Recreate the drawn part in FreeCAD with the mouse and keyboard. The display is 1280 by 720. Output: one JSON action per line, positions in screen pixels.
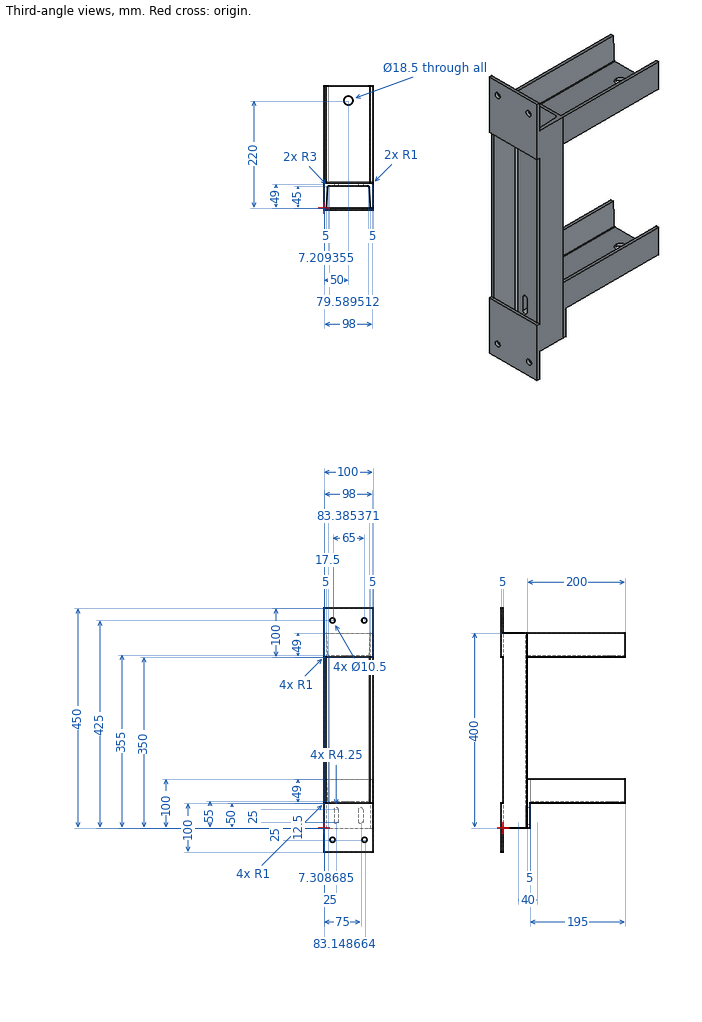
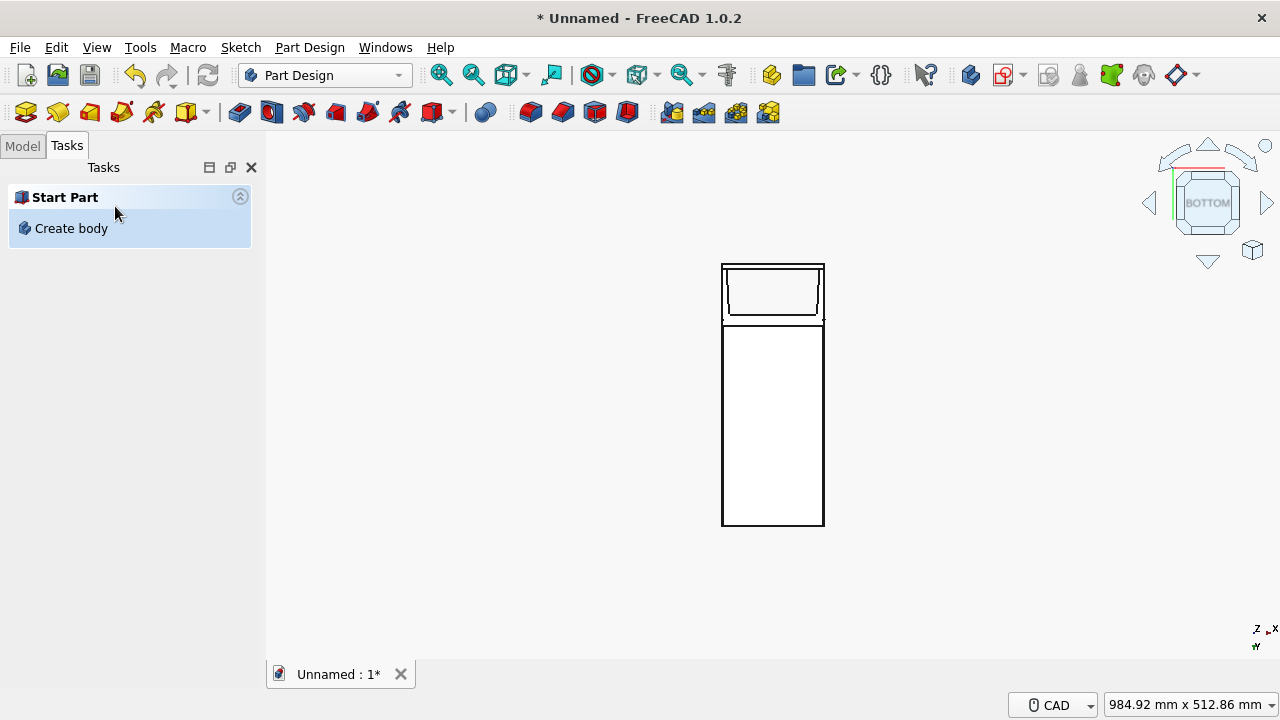
{"action": "left_click", "coordinate": [773, 454]}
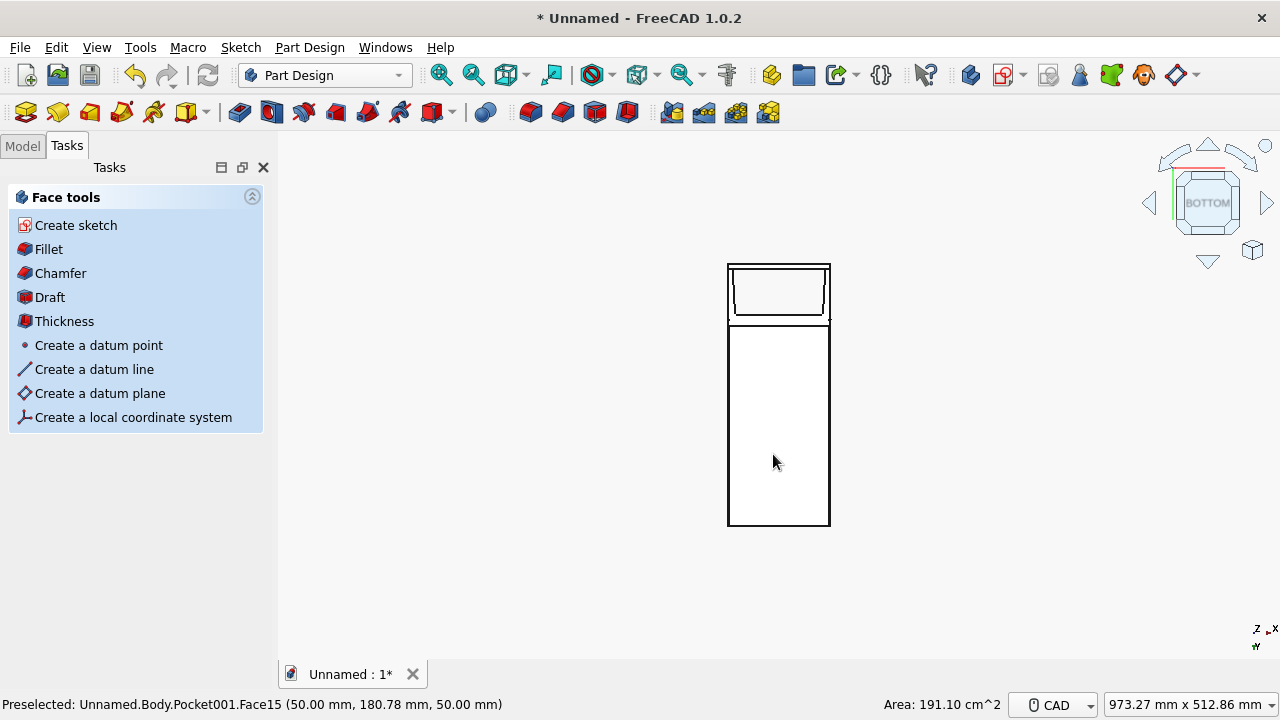
{"action": "left_click", "coordinate": [1004, 76]}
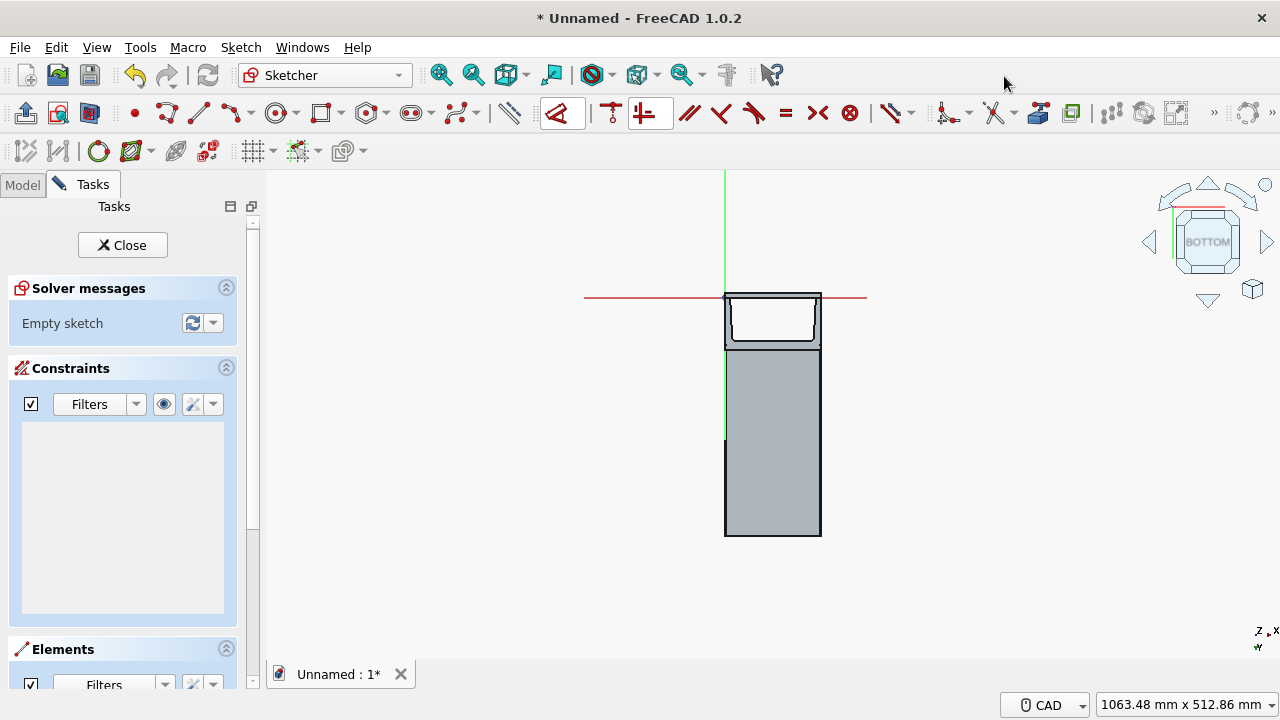
{"action": "key", "text": "q s"}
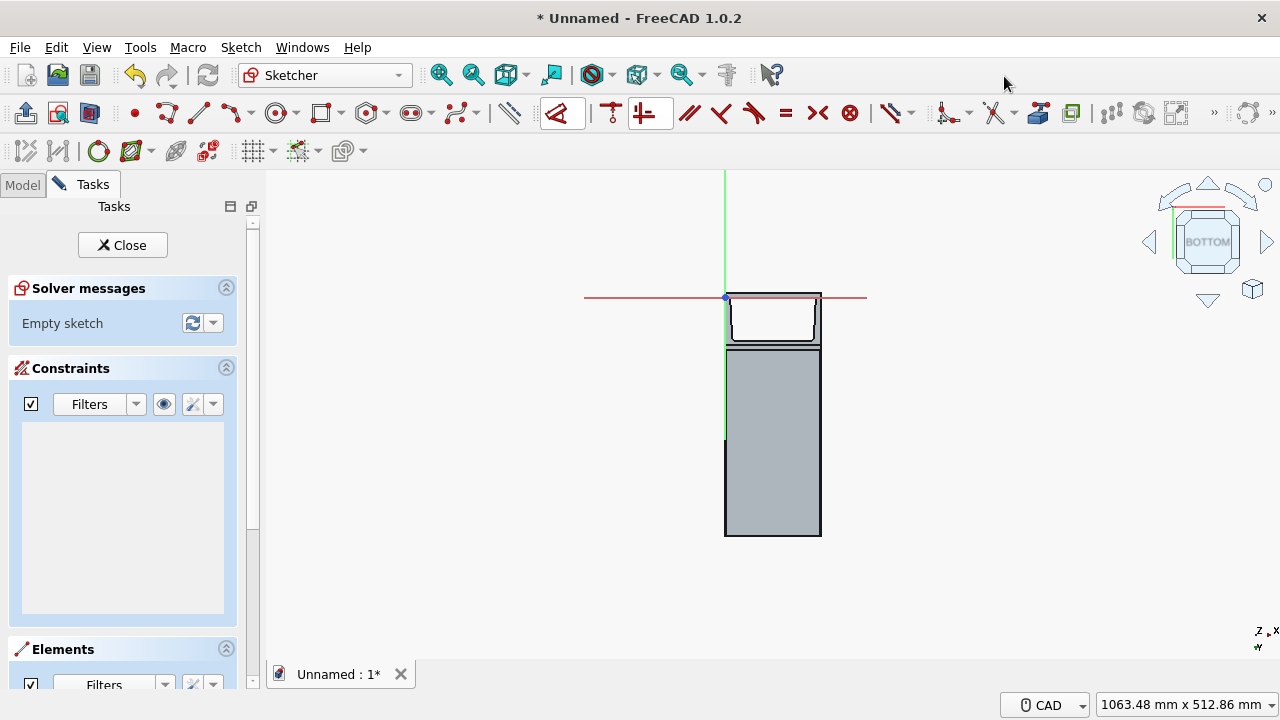
{"action": "scroll", "coordinate": [777, 513], "scroll_direction": "up", "scroll_amount": 14}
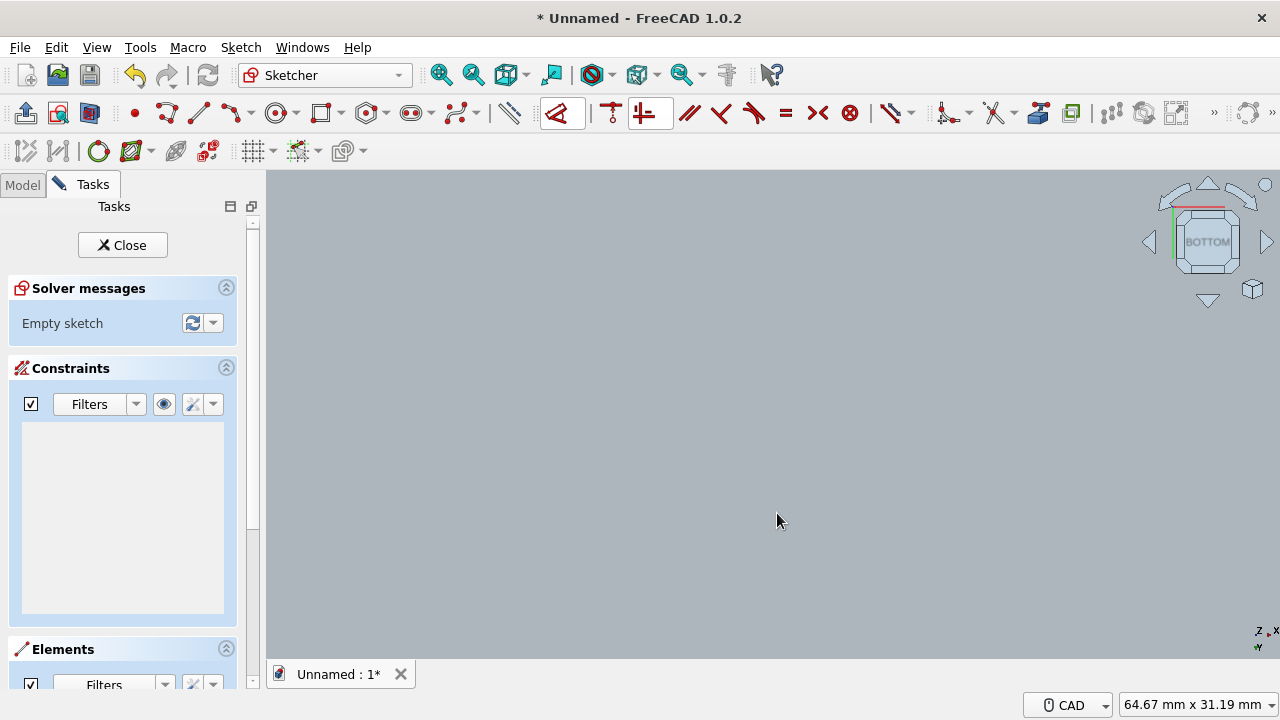
{"action": "left_click", "coordinate": [276, 114]}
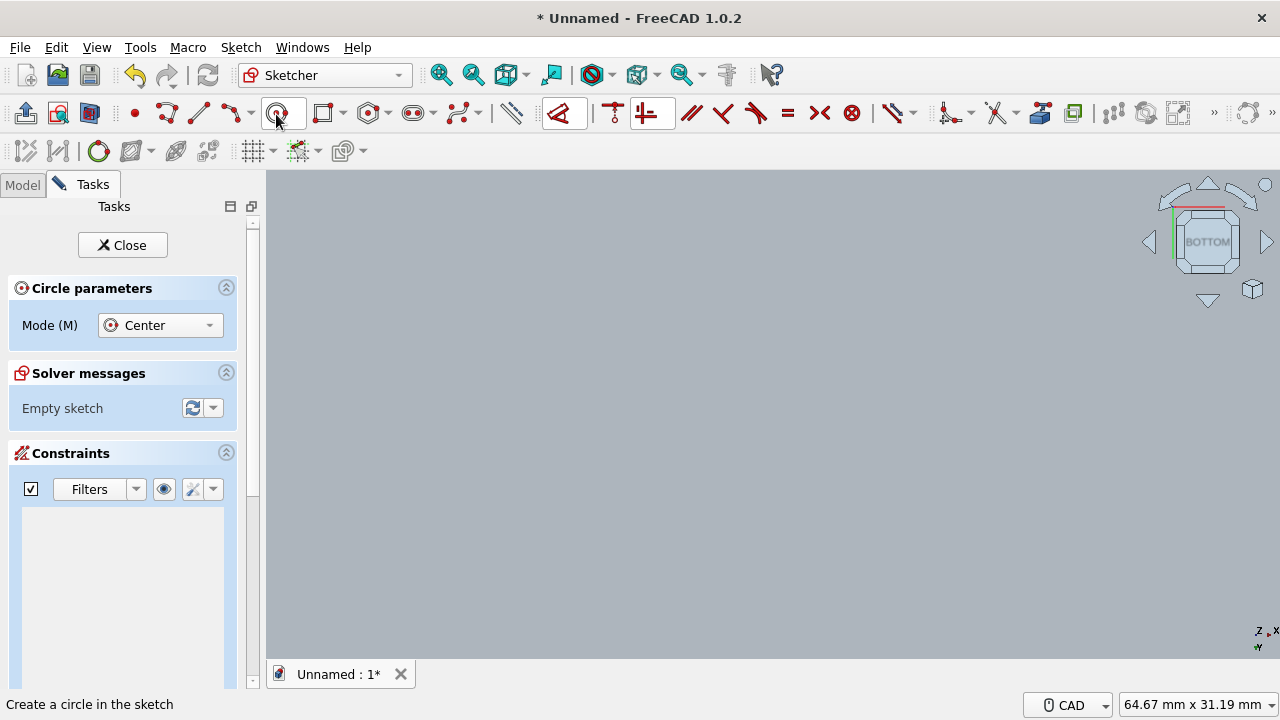
{"action": "left_click", "coordinate": [703, 411]}
{"action": "left_click", "coordinate": [806, 309]}
{"action": "key", "text": "Escape"}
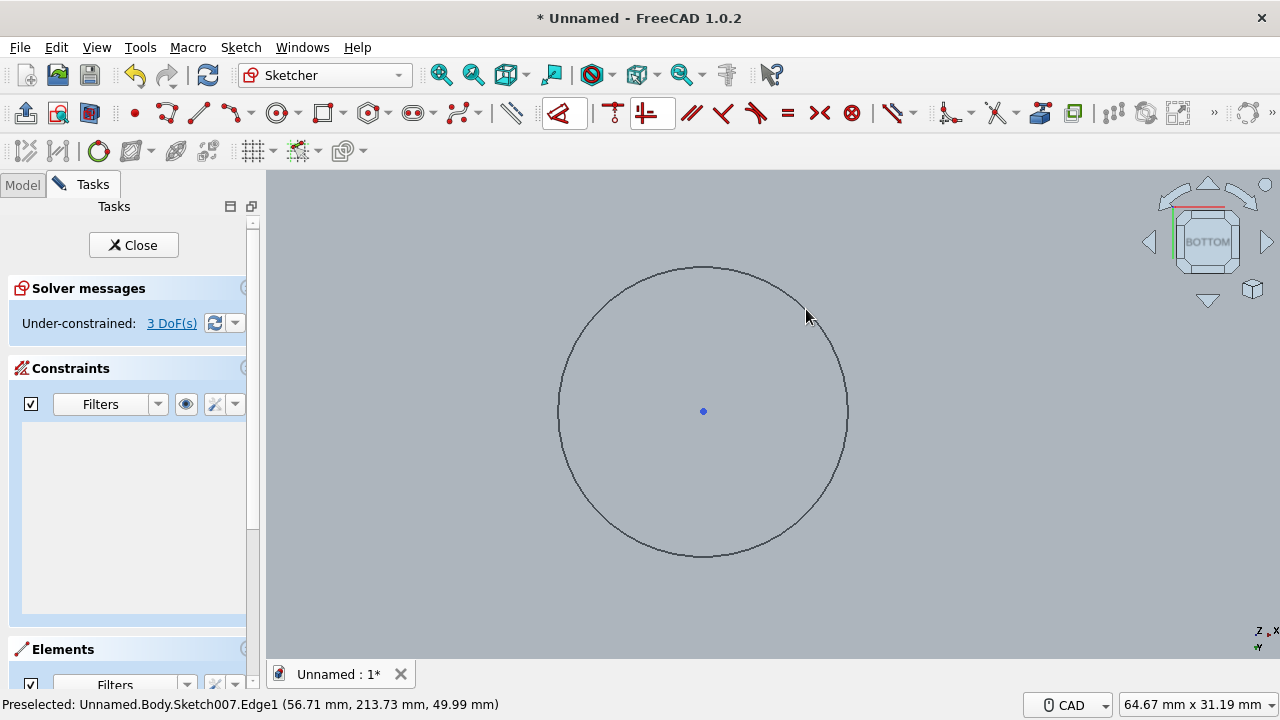
{"action": "left_click", "coordinate": [805, 309]}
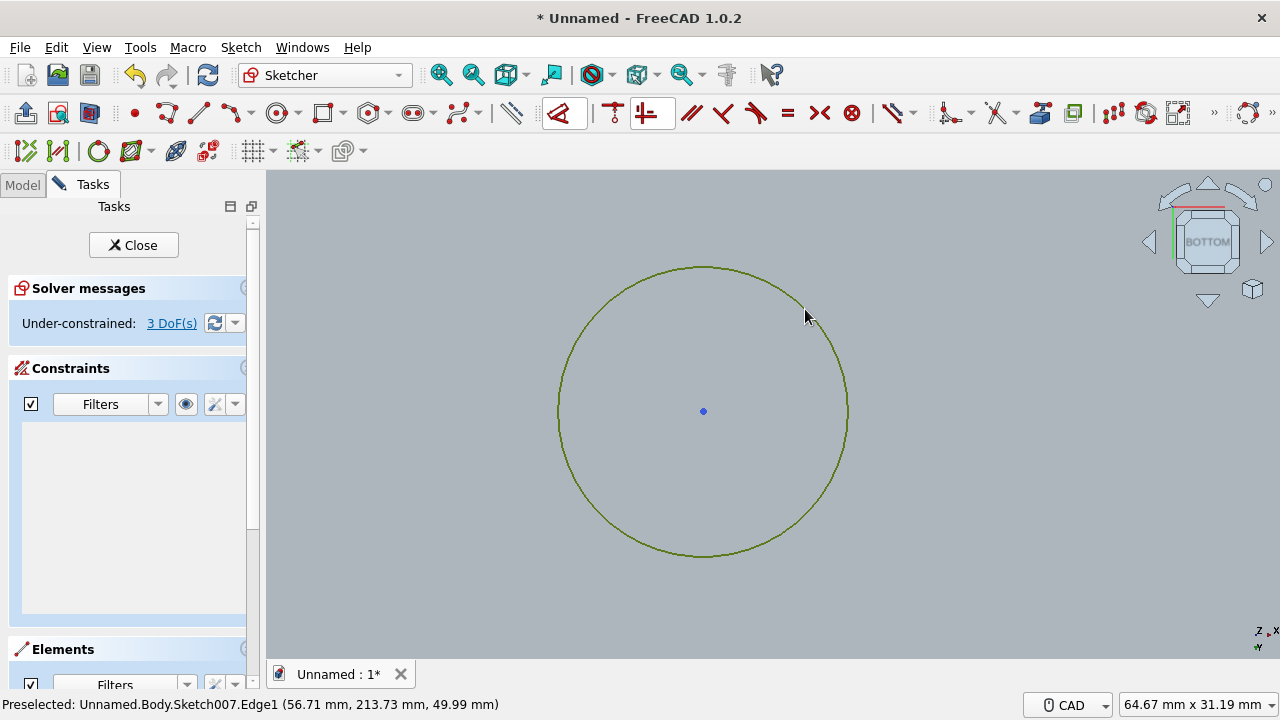
{"action": "key", "text": "k o"}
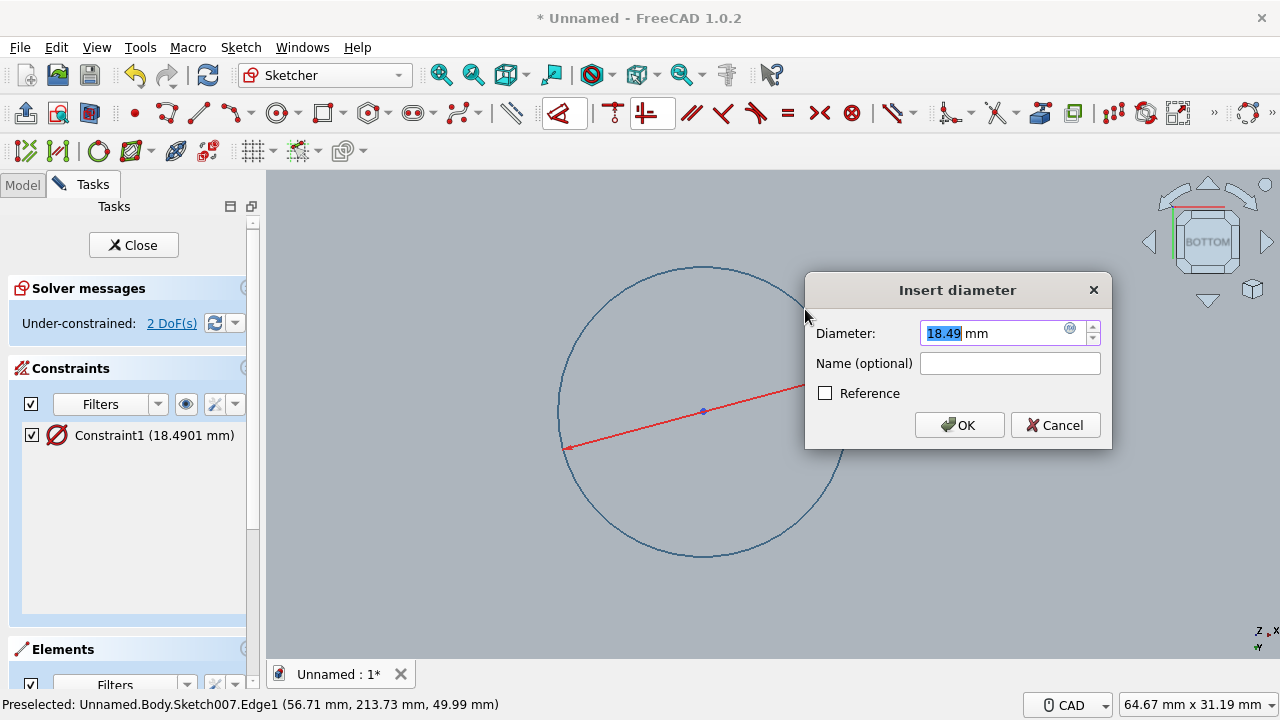
{"action": "type", "text": "18.5"}
{"action": "key", "text": "Return"}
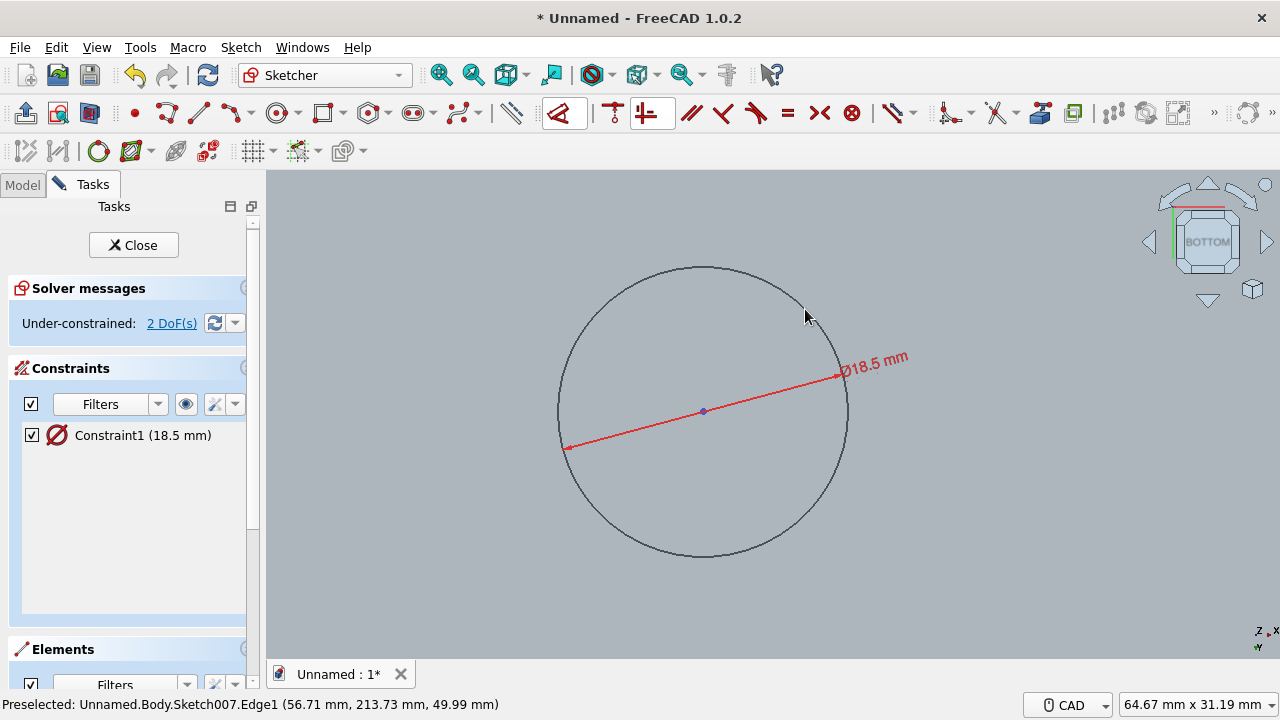
{"action": "left_click", "coordinate": [703, 412]}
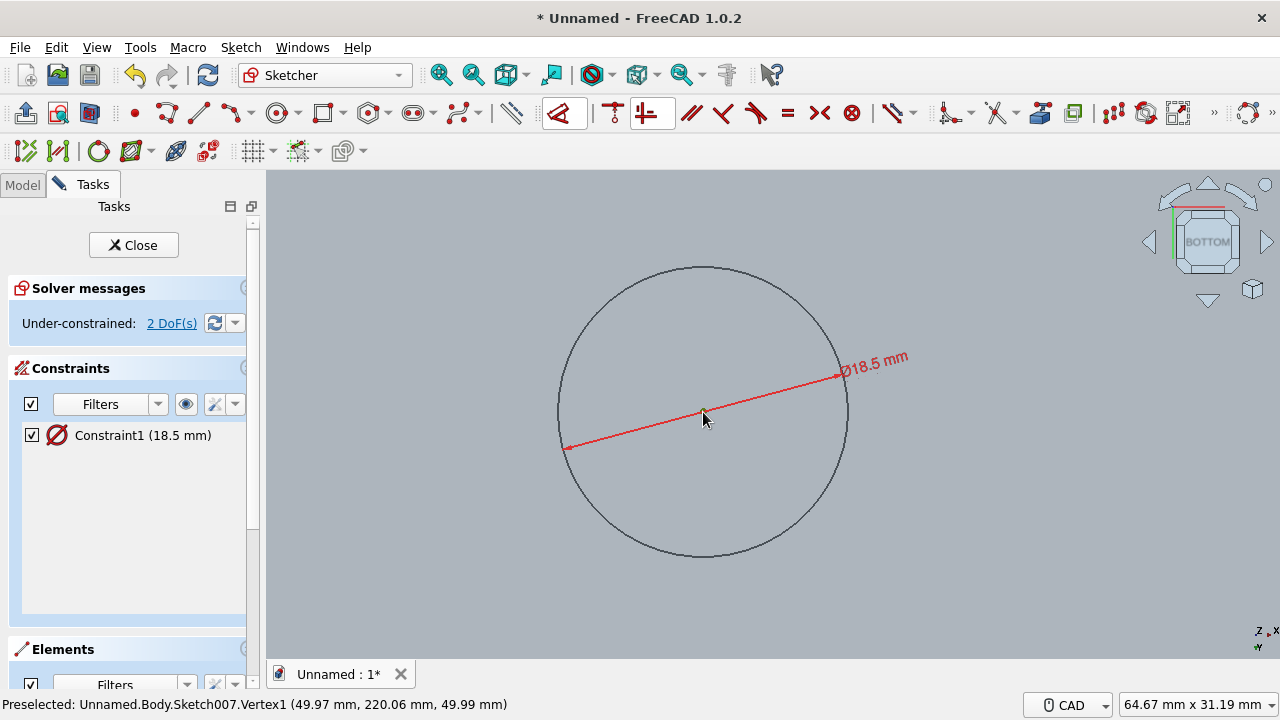
{"action": "left_click", "coordinate": [582, 114]}